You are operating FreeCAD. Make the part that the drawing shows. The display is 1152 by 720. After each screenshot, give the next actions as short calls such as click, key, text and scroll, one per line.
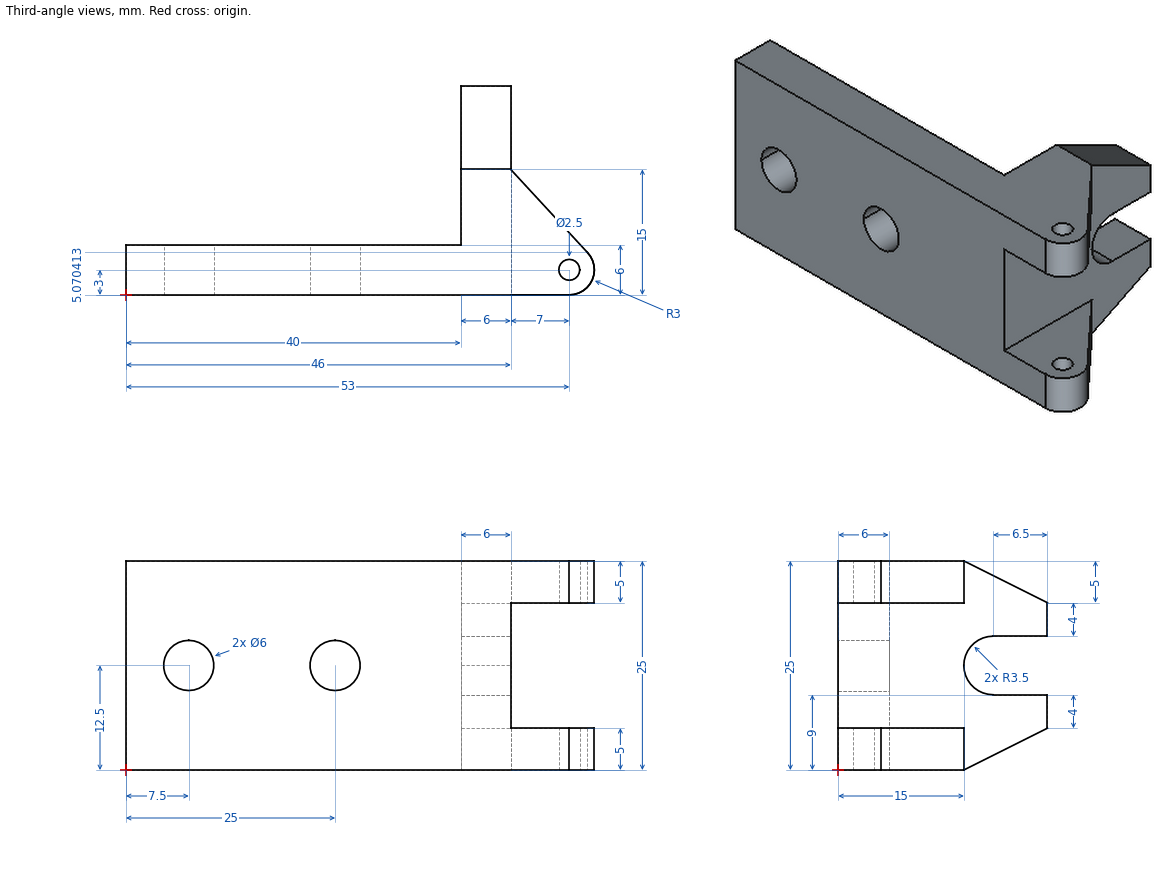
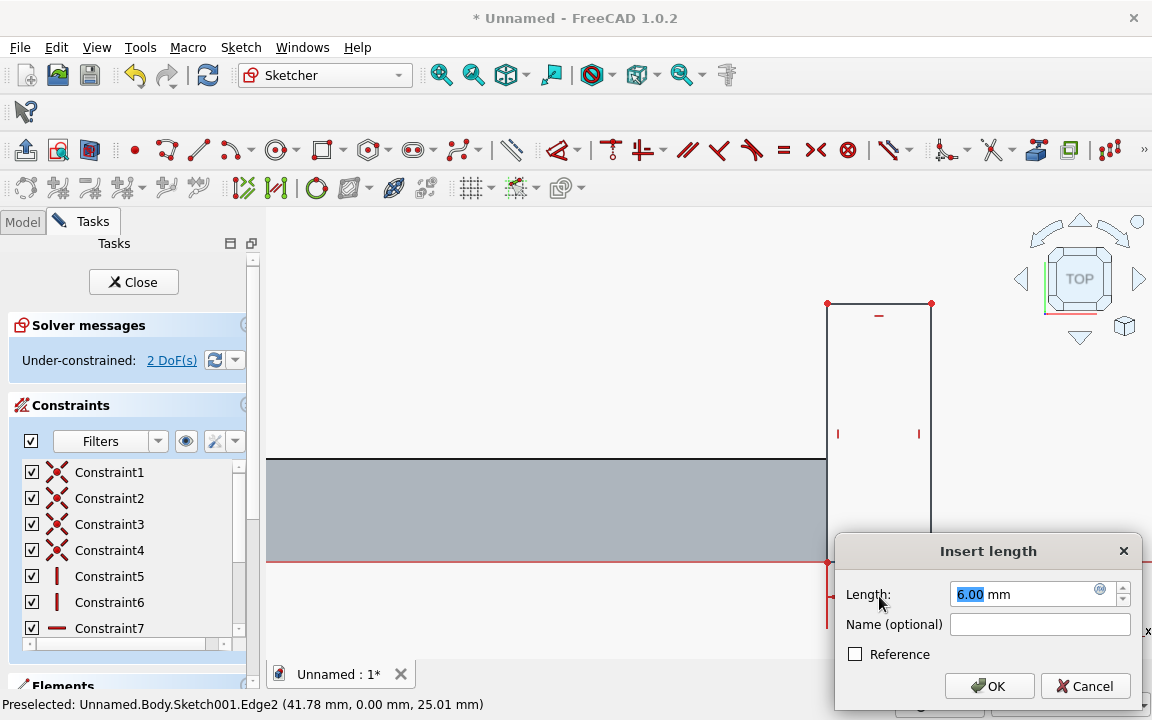
text(6)
key(Return)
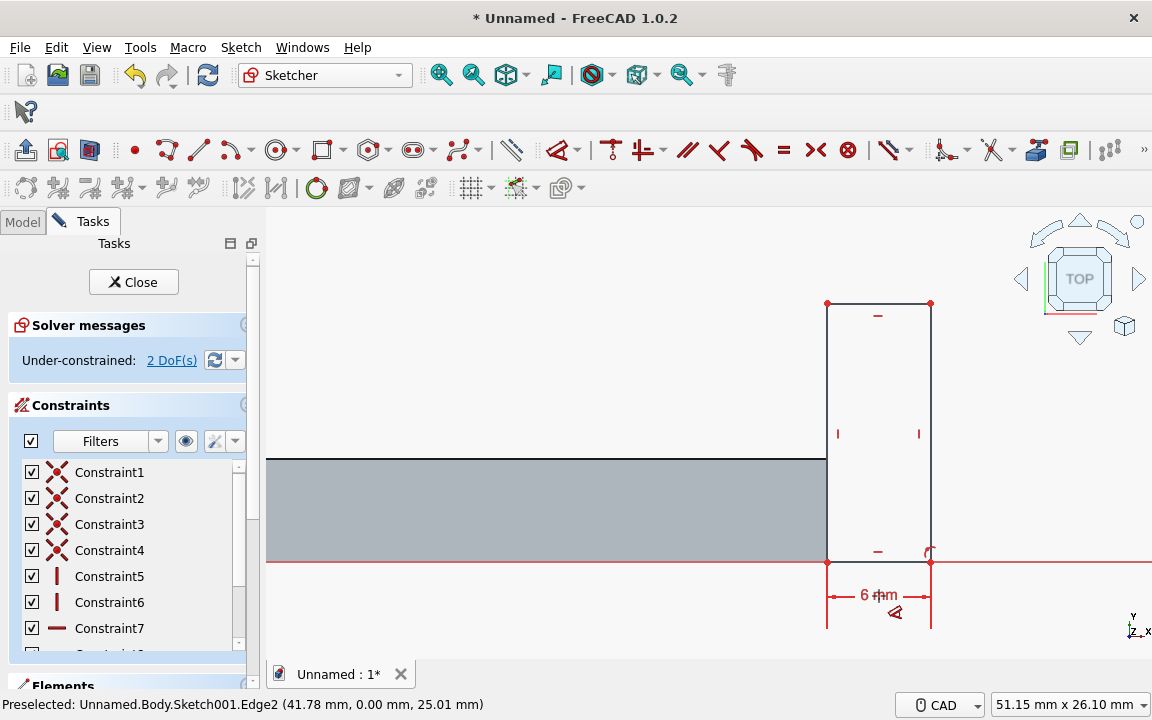
click(827, 382)
click(793, 433)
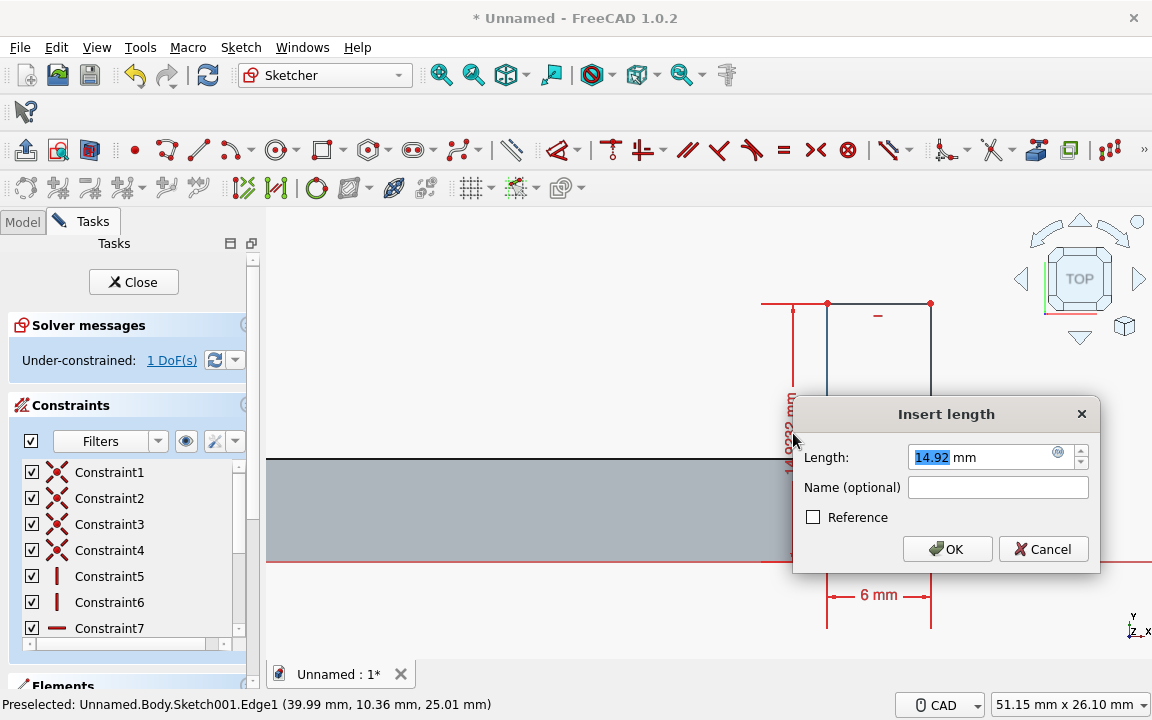
text(15)
key(Return)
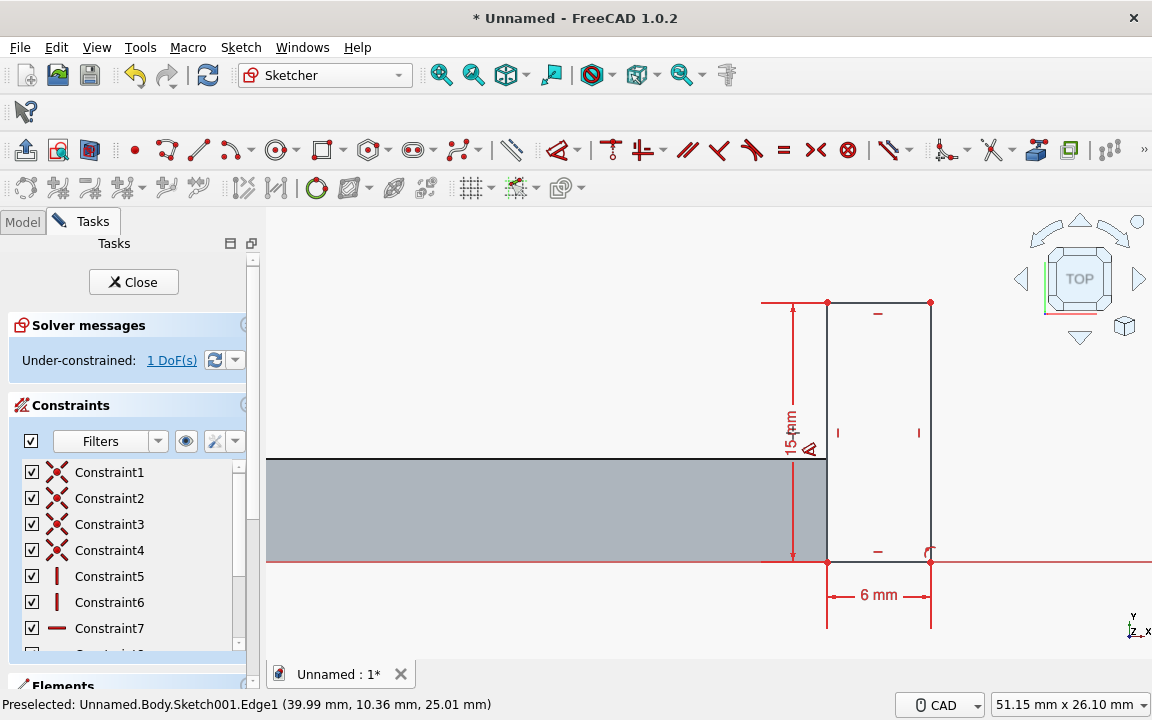
click(827, 303)
click(561, 596)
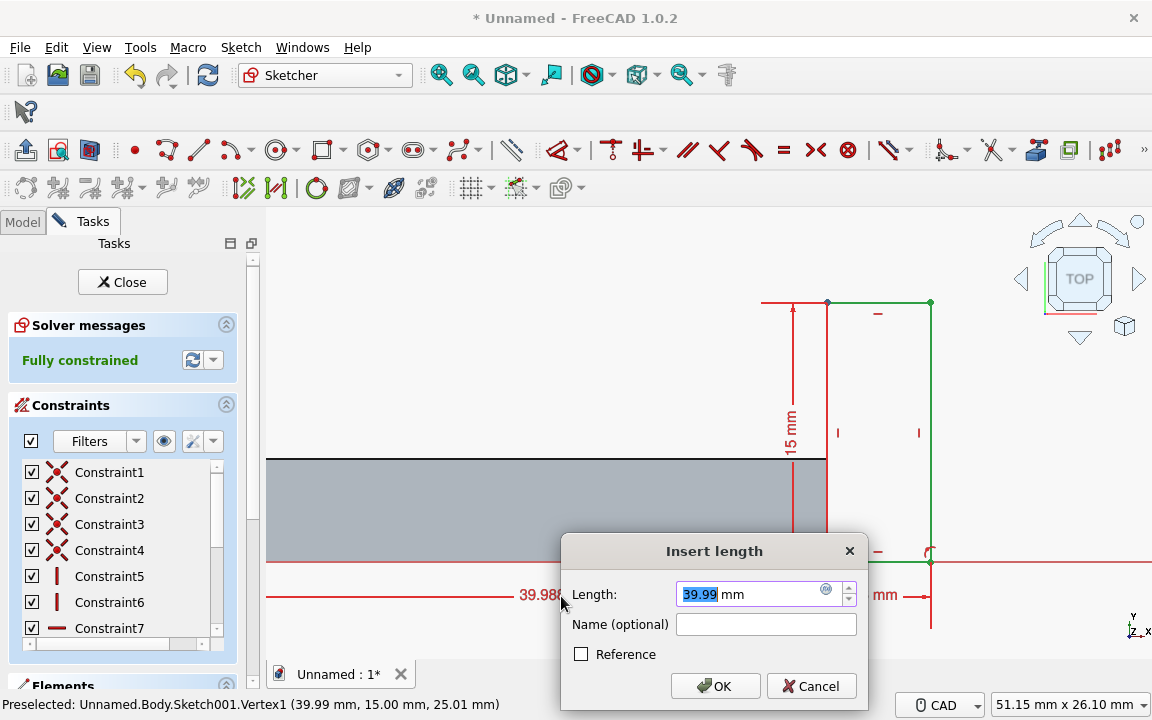
text(40)
key(Return)
key(Escape)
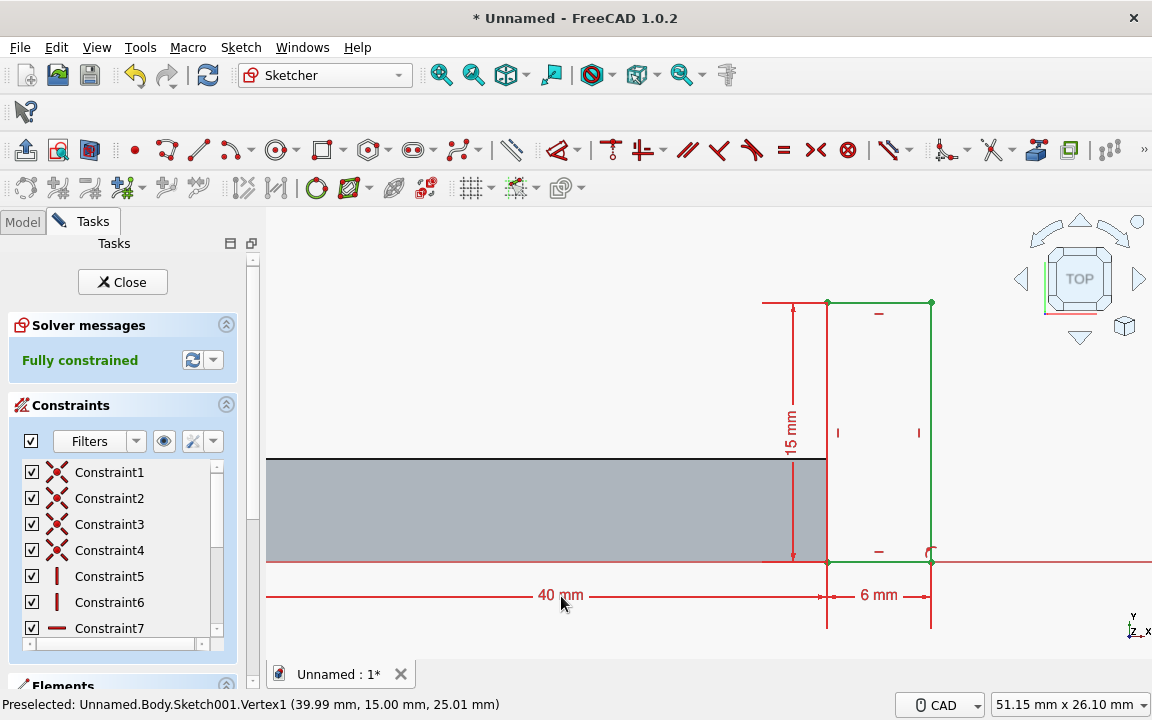
click(123, 282)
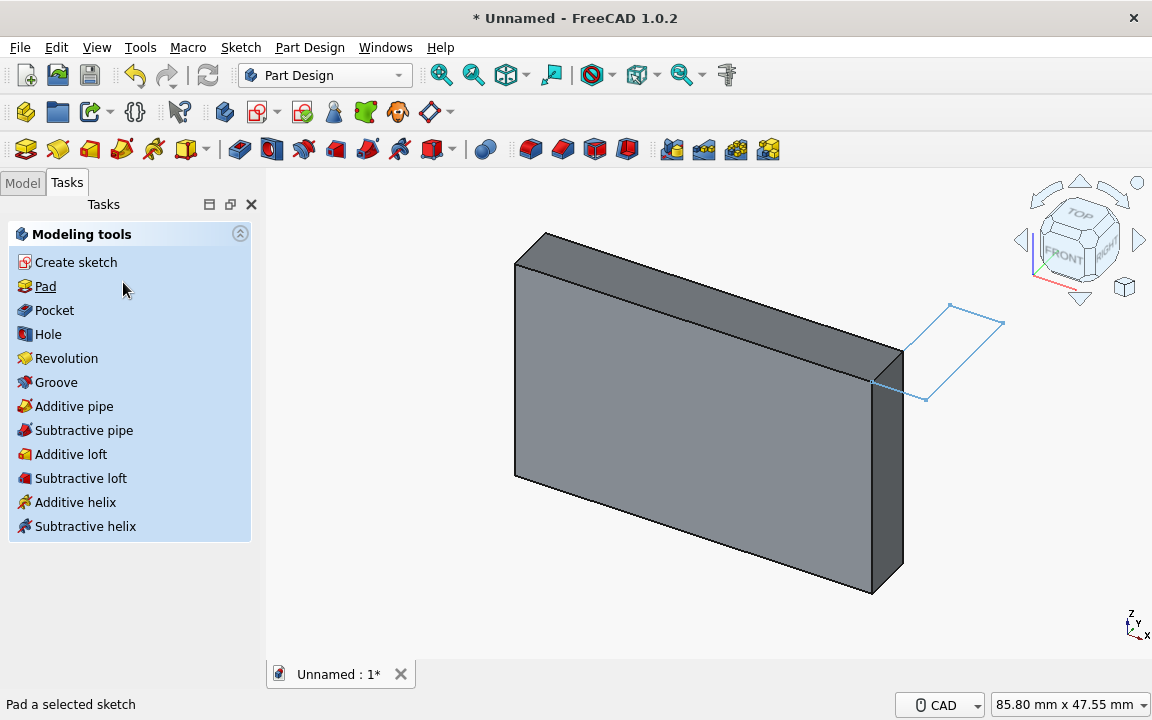
click(26, 150)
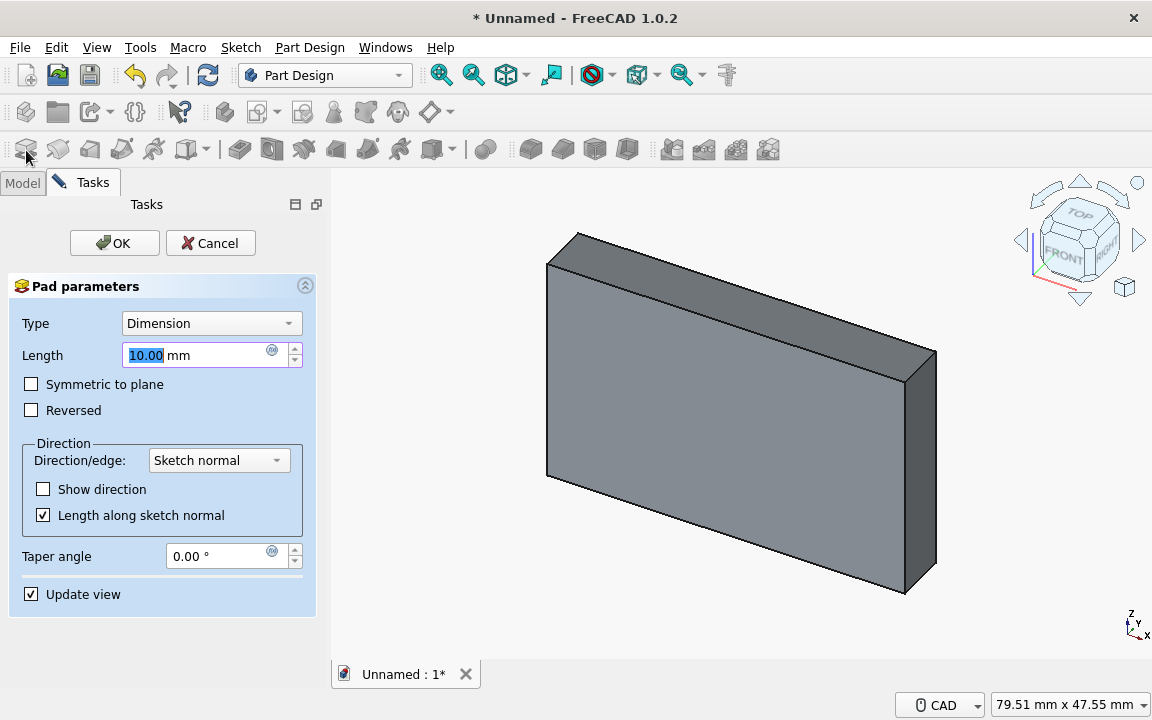
text(25)
key(Tab)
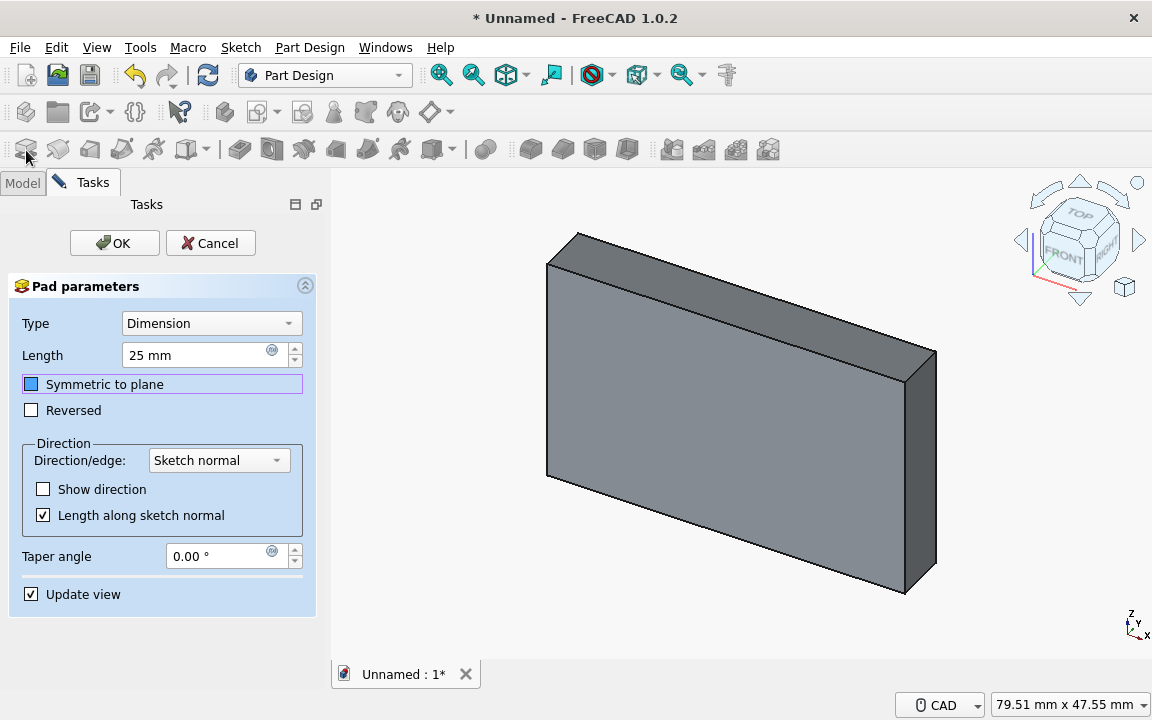
click(30, 410)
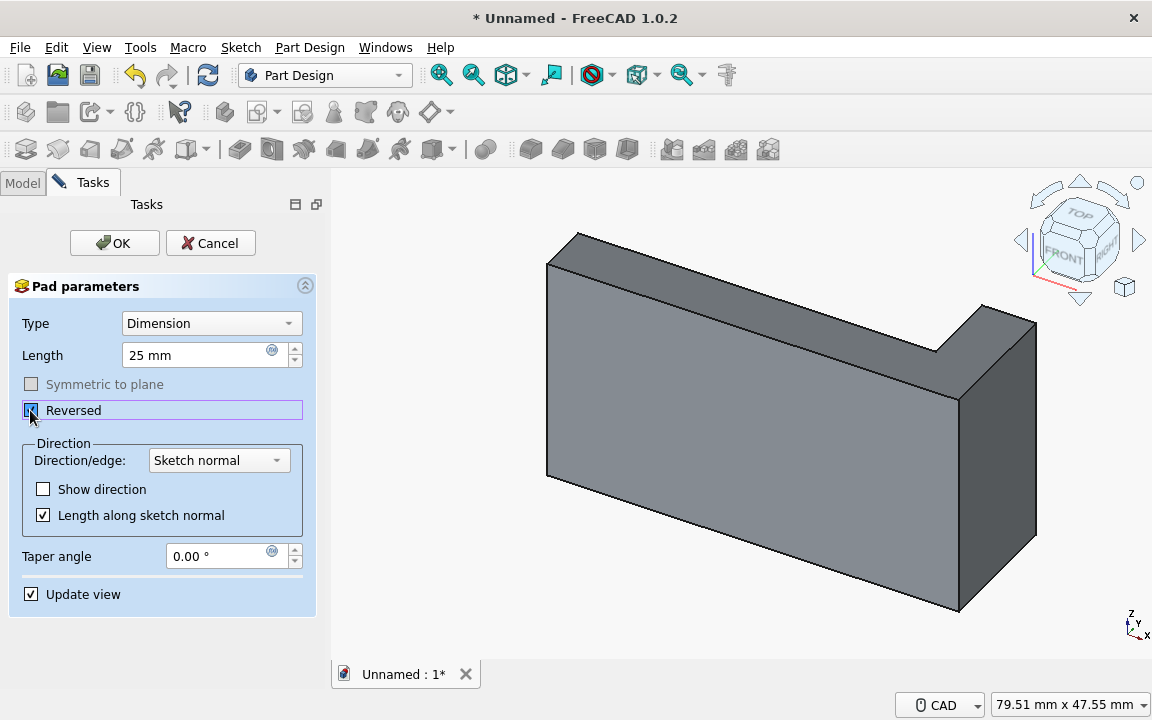
click(115, 243)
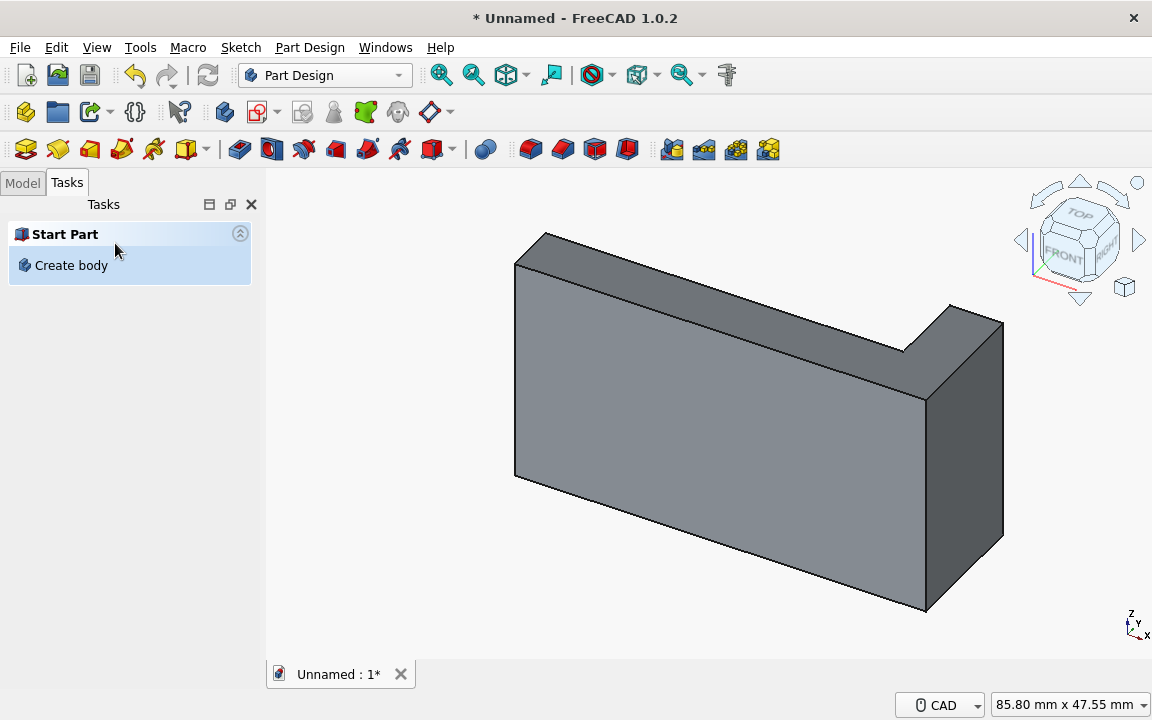
key(6)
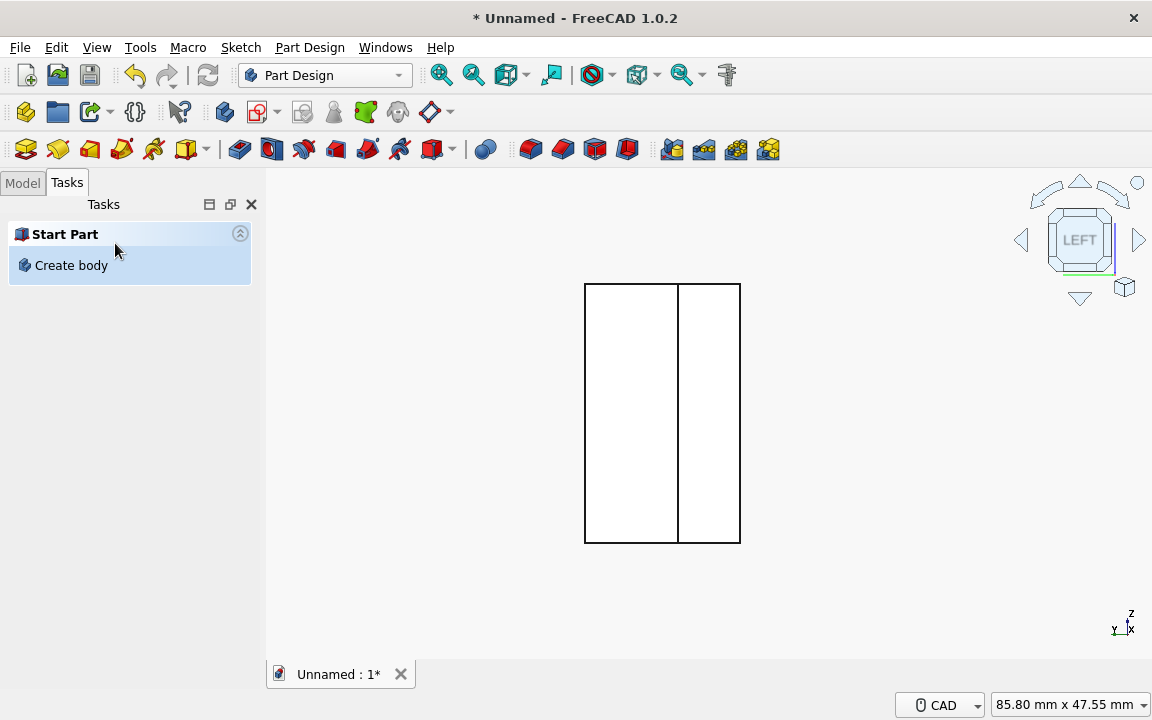
click(632, 339)